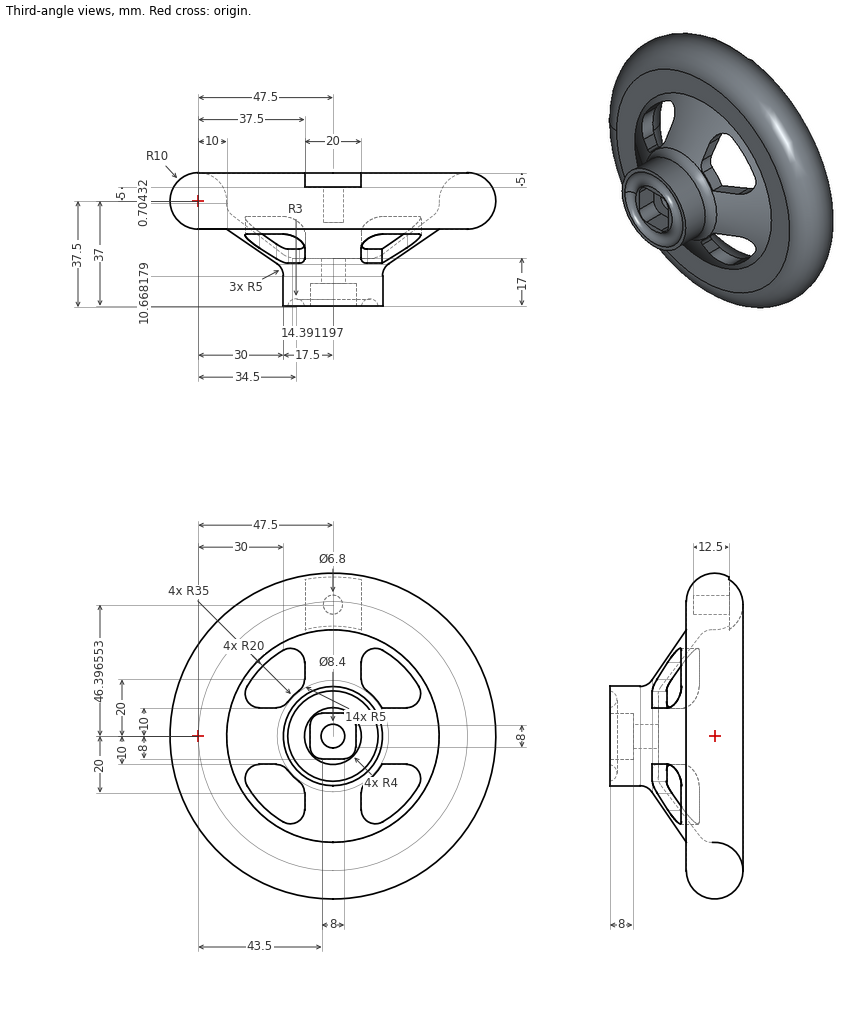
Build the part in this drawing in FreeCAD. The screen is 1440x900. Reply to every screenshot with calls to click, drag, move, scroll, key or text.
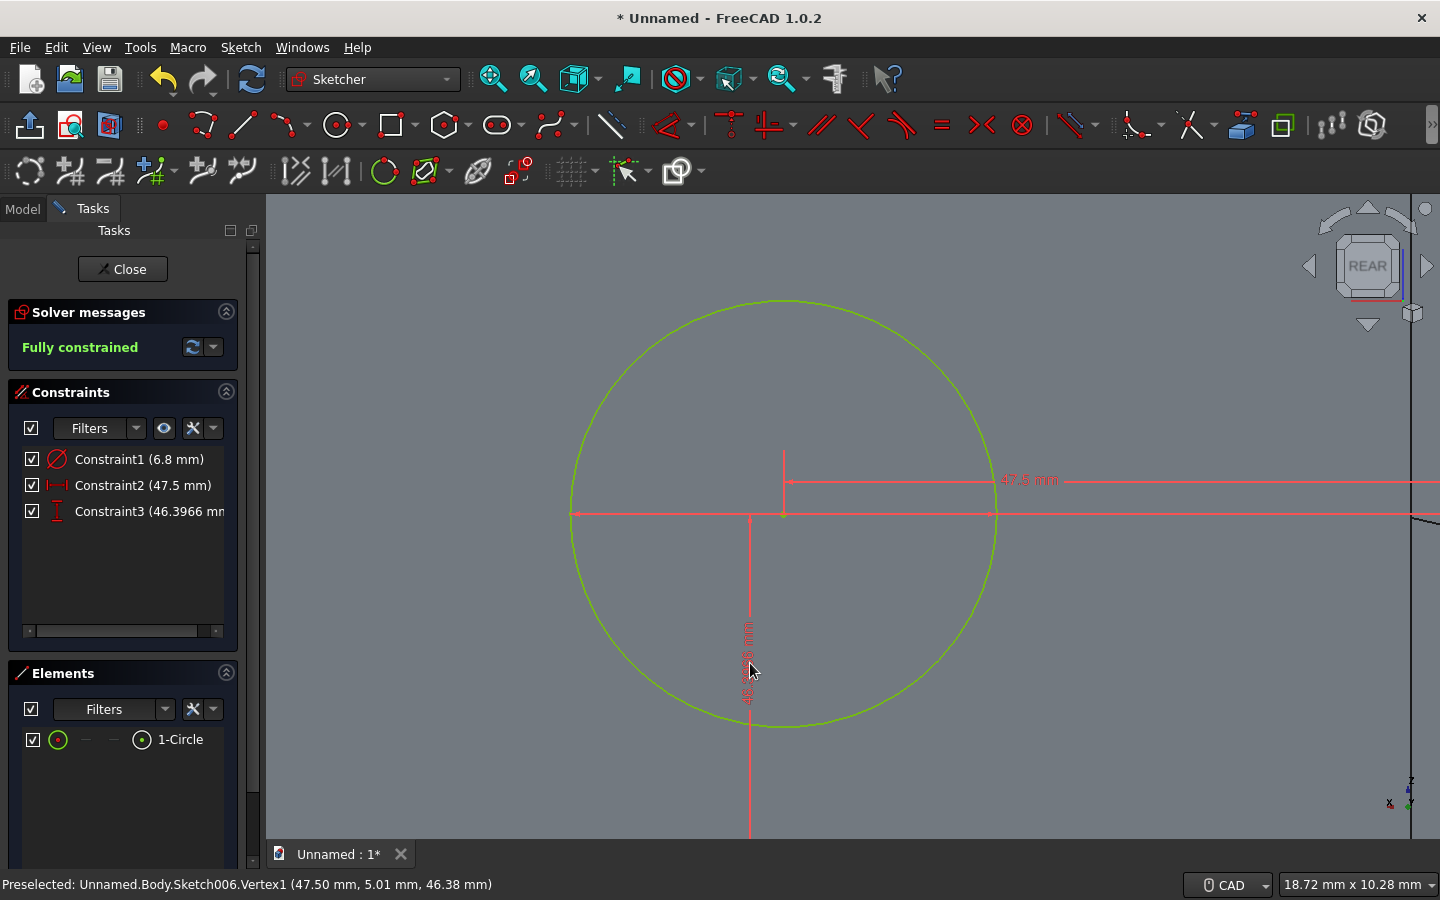
click(123, 269)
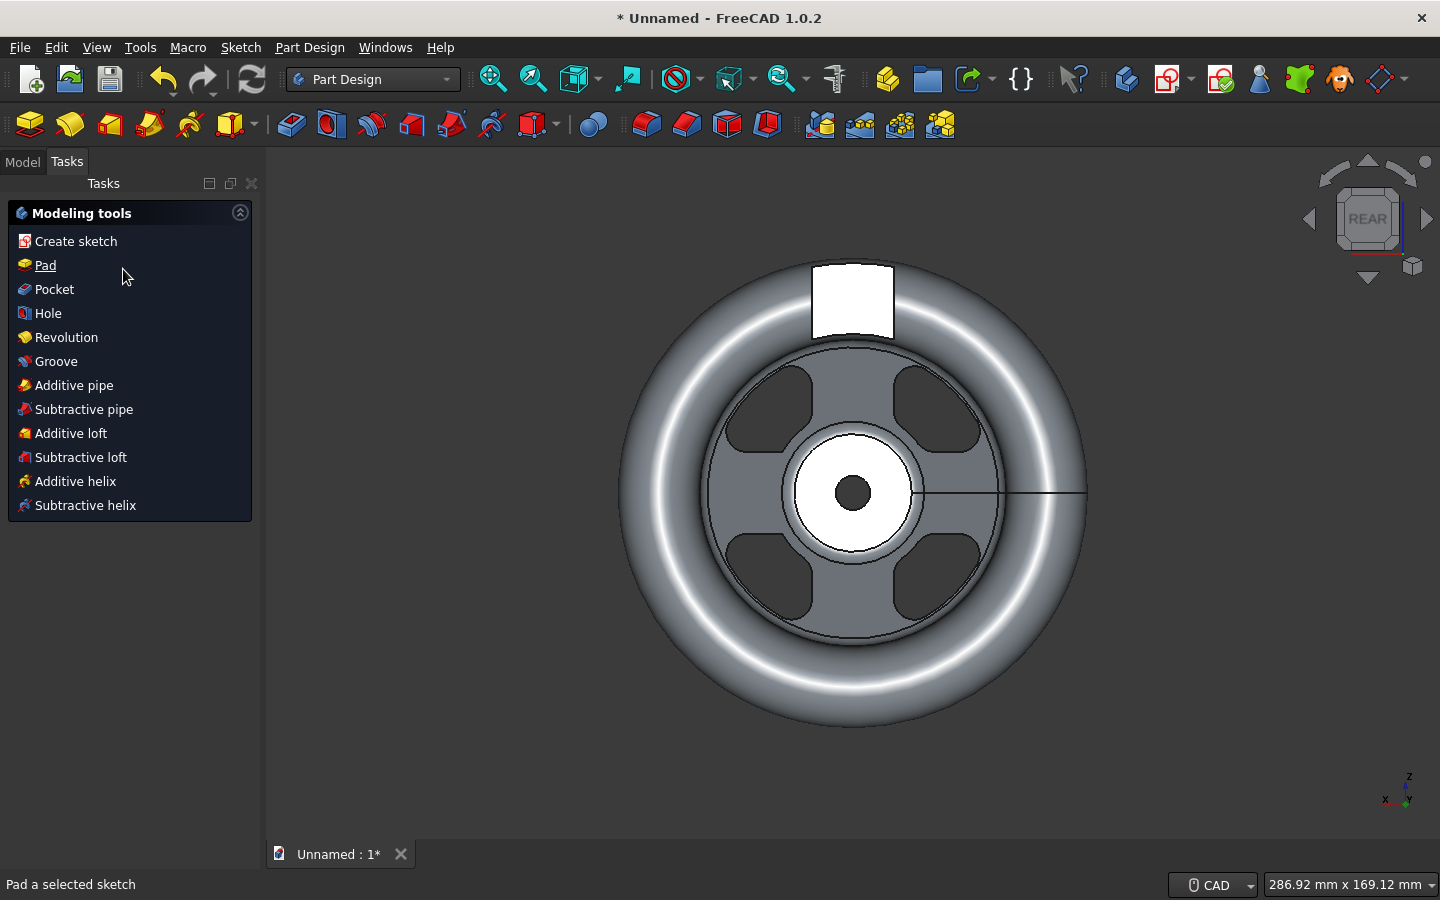
click(292, 124)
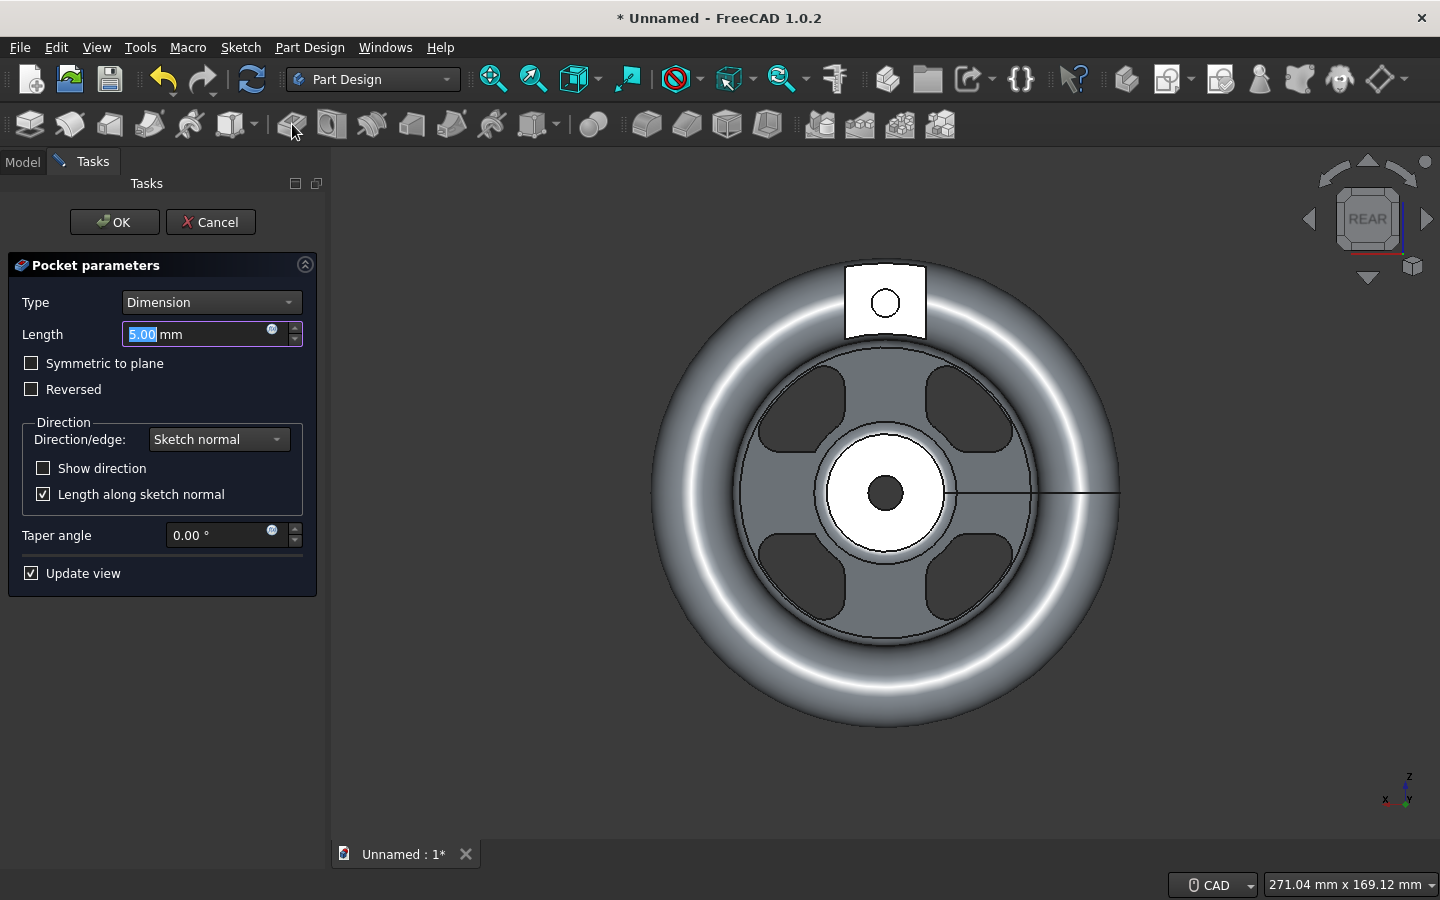
text(12.5)
key(Tab)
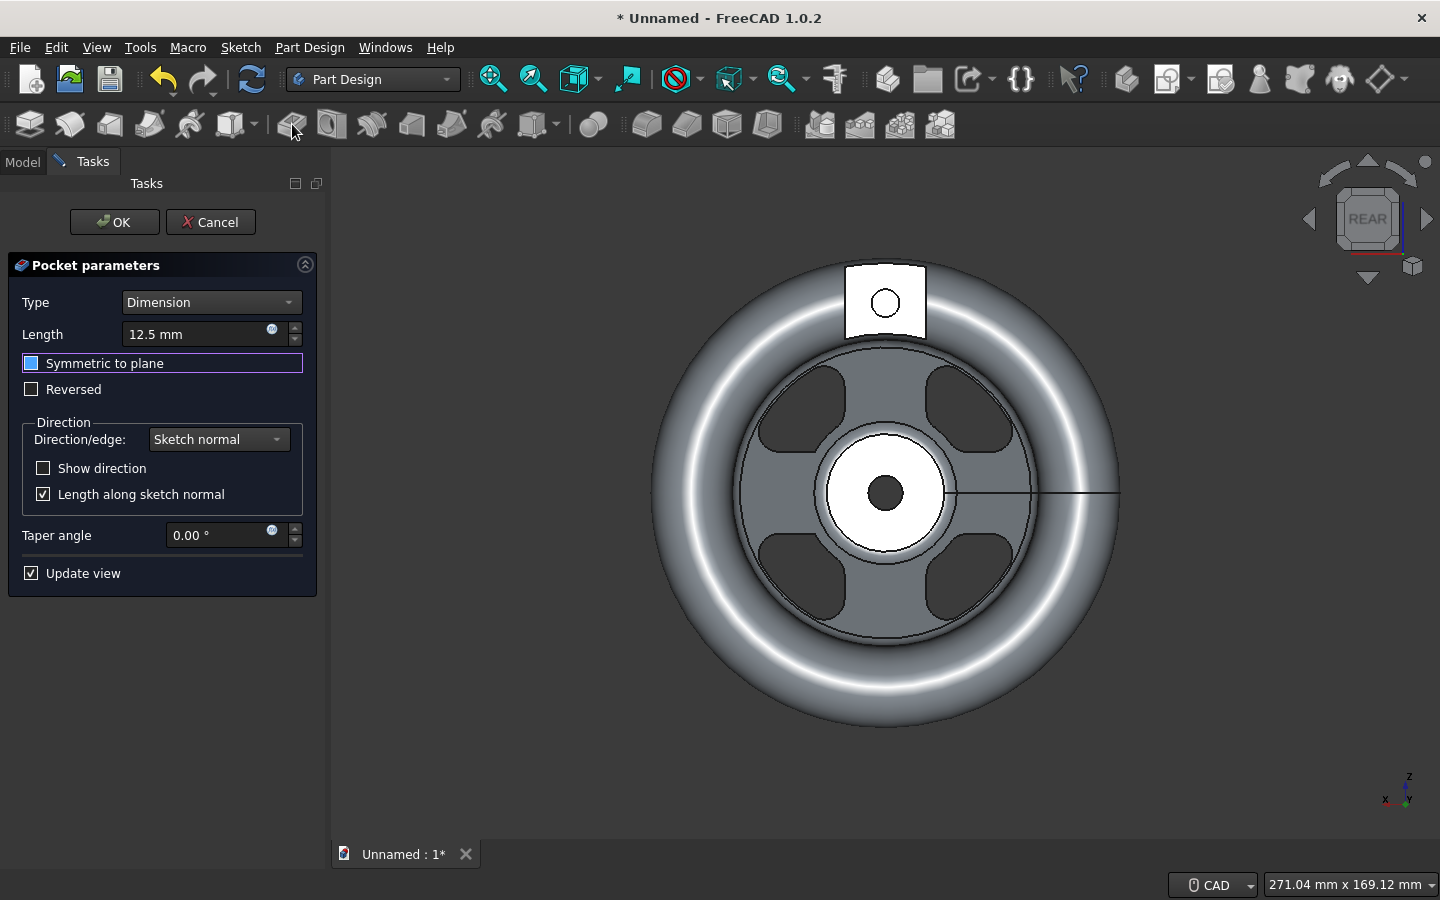
click(115, 222)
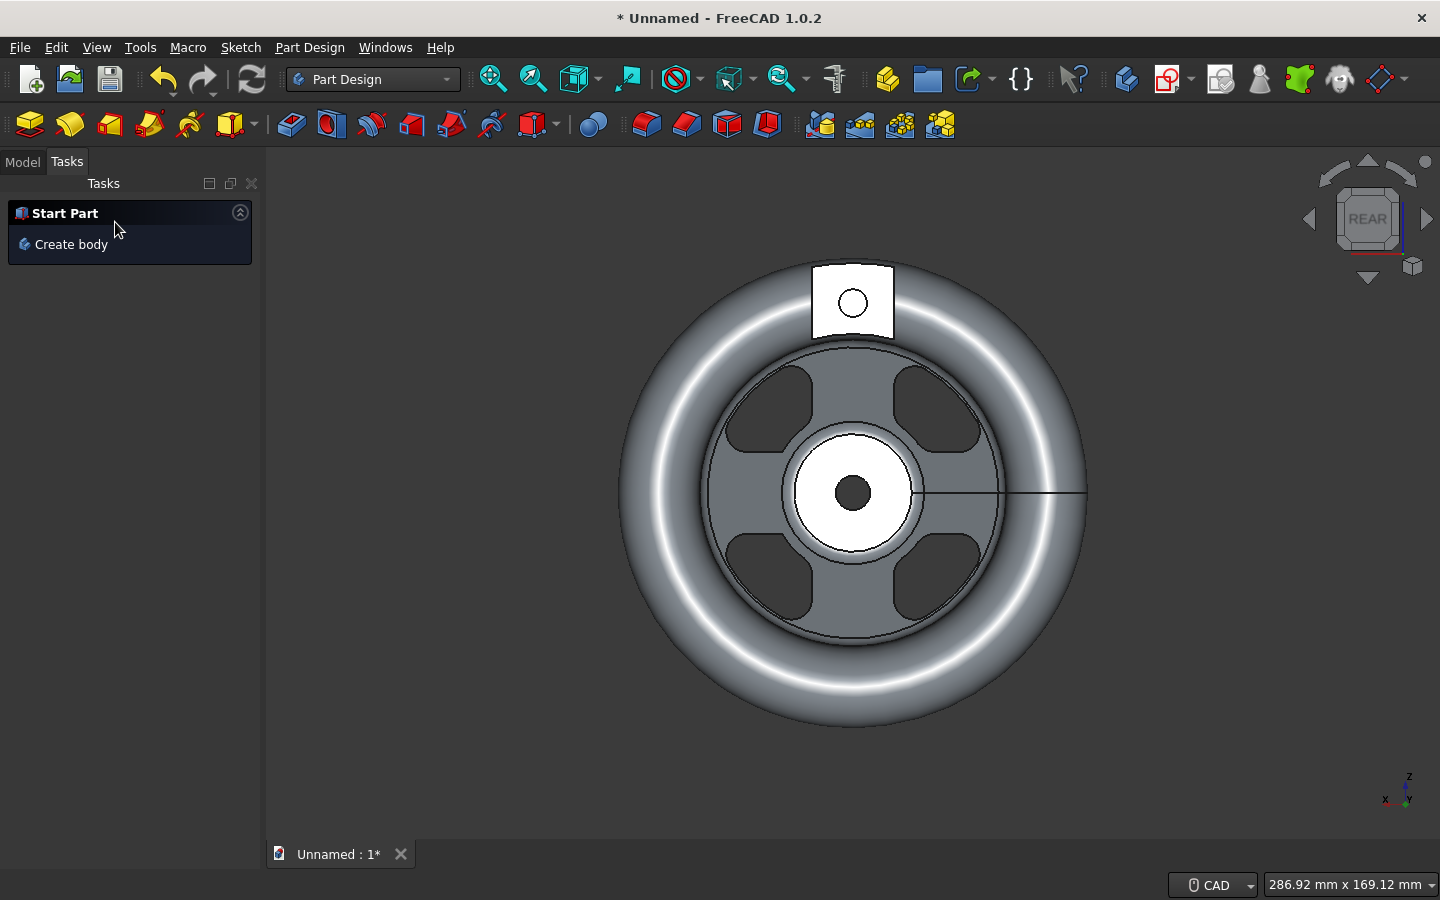
key(0)